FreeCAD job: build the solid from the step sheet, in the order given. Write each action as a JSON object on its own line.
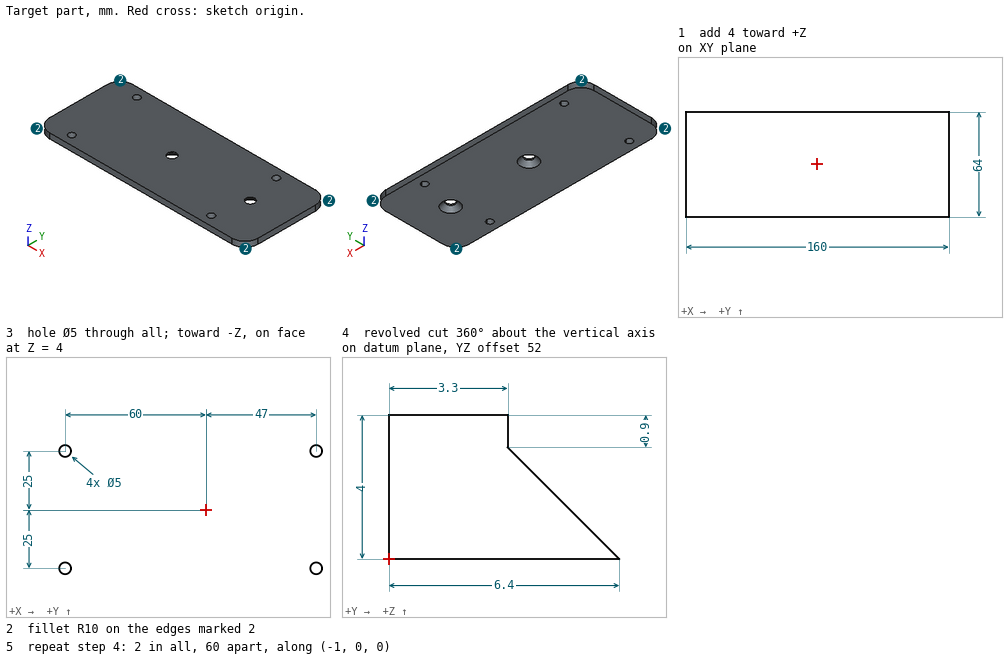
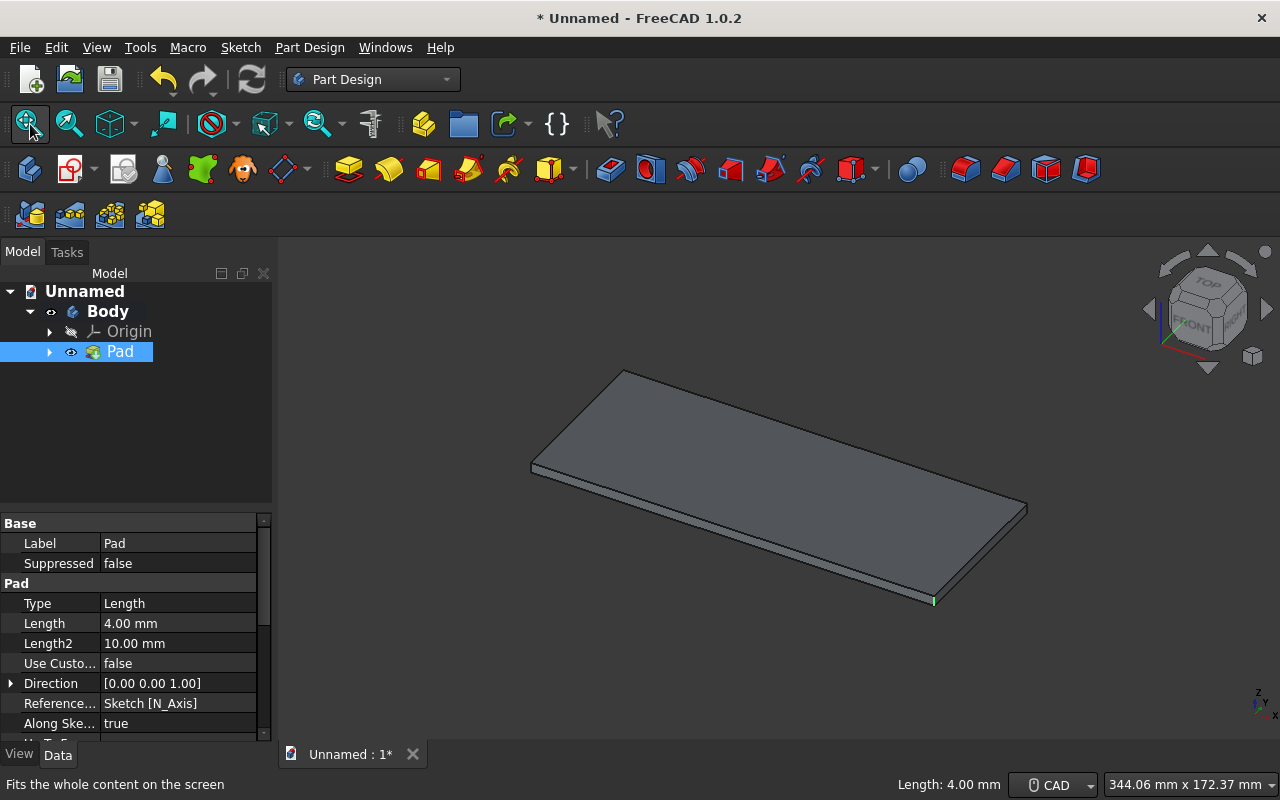
{"action": "key", "text": "0"}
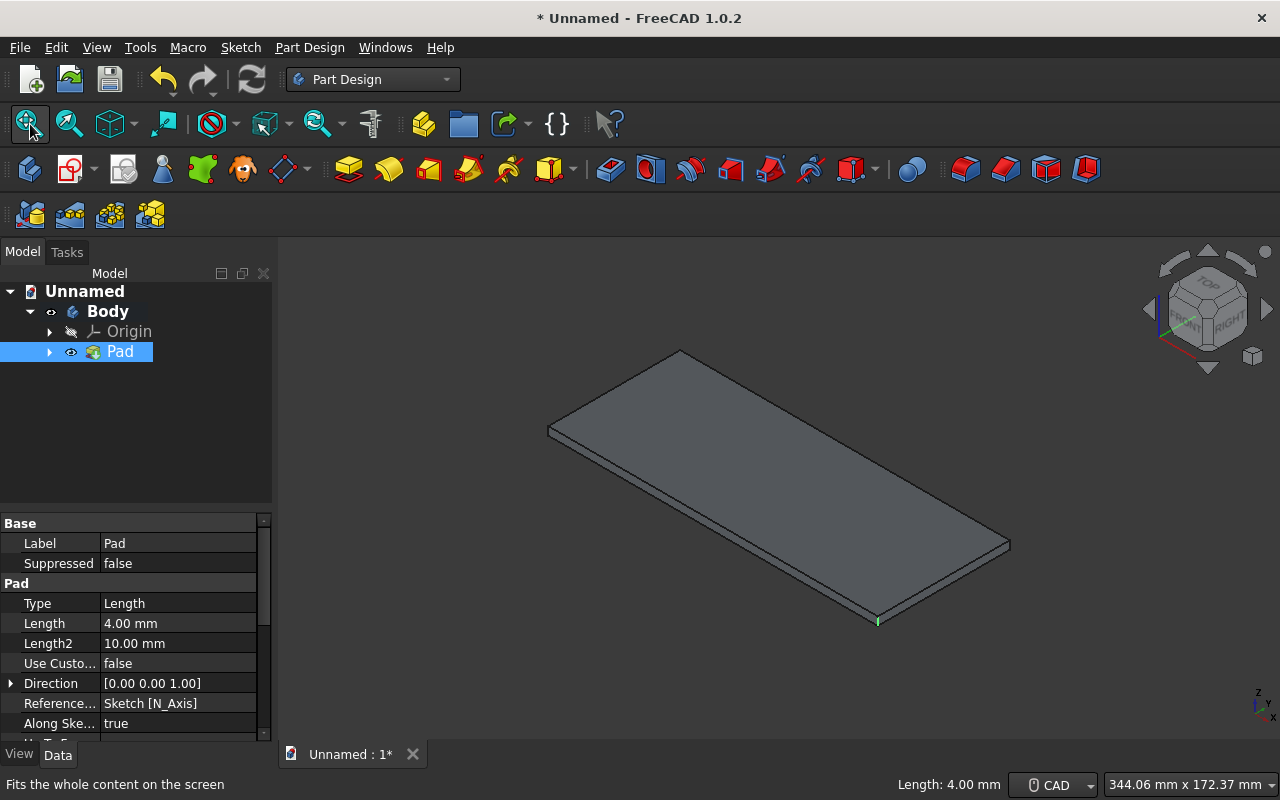
{"action": "scroll", "coordinate": [548, 430], "scroll_direction": "up", "scroll_amount": 7}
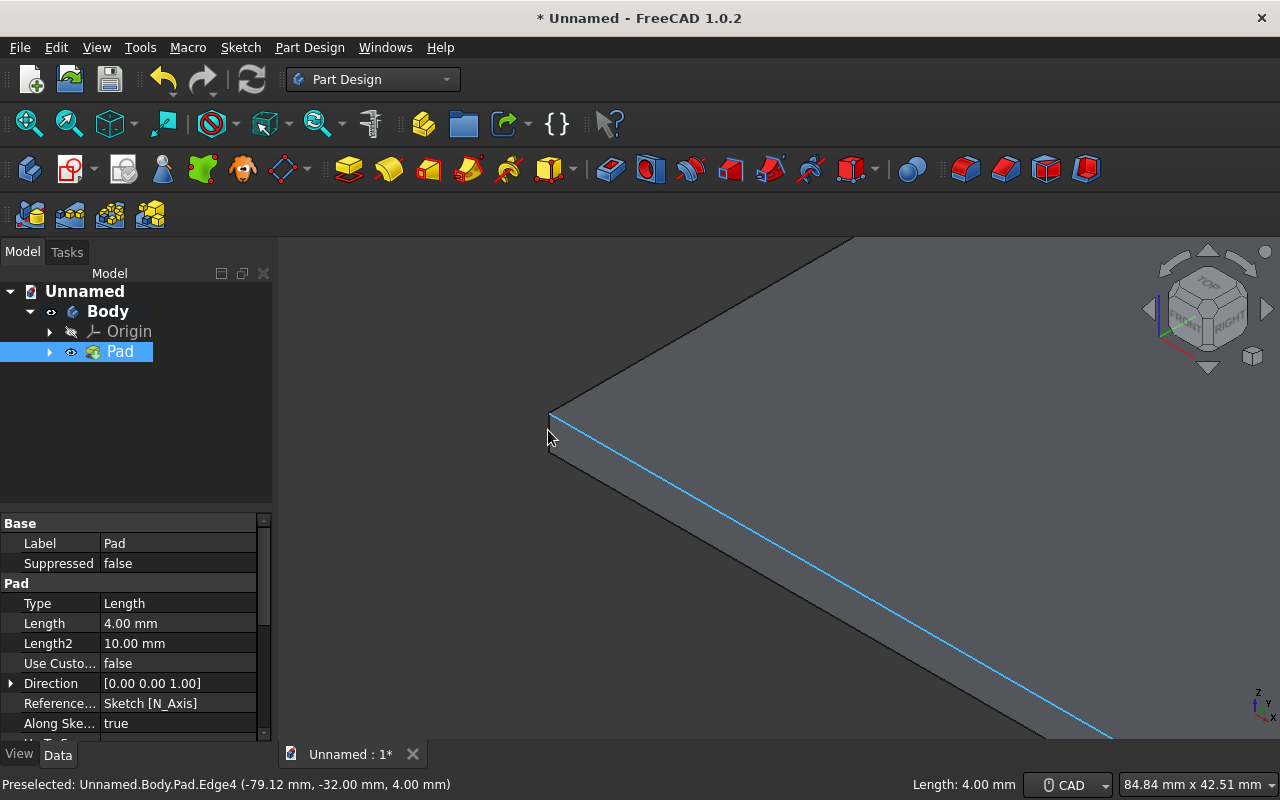
{"action": "left_click", "coordinate": [30, 124]}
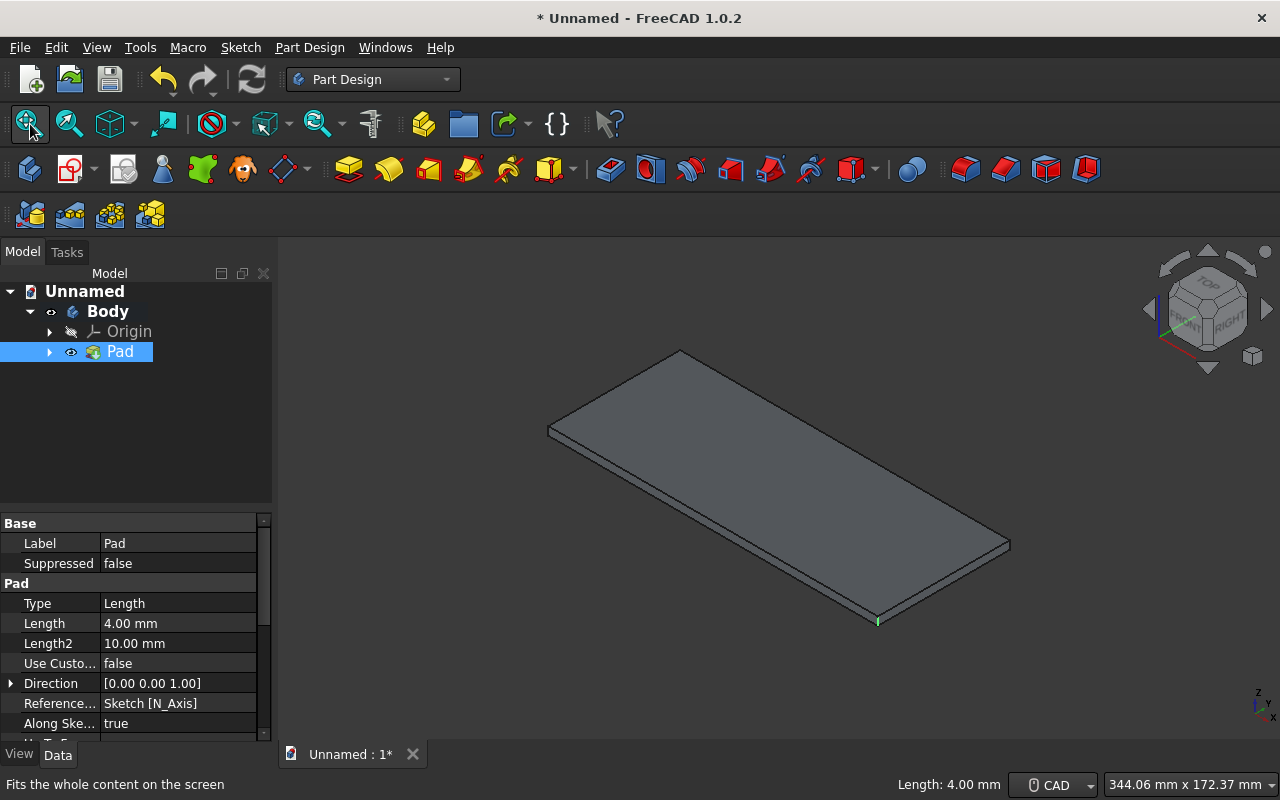
{"action": "key", "text": "2"}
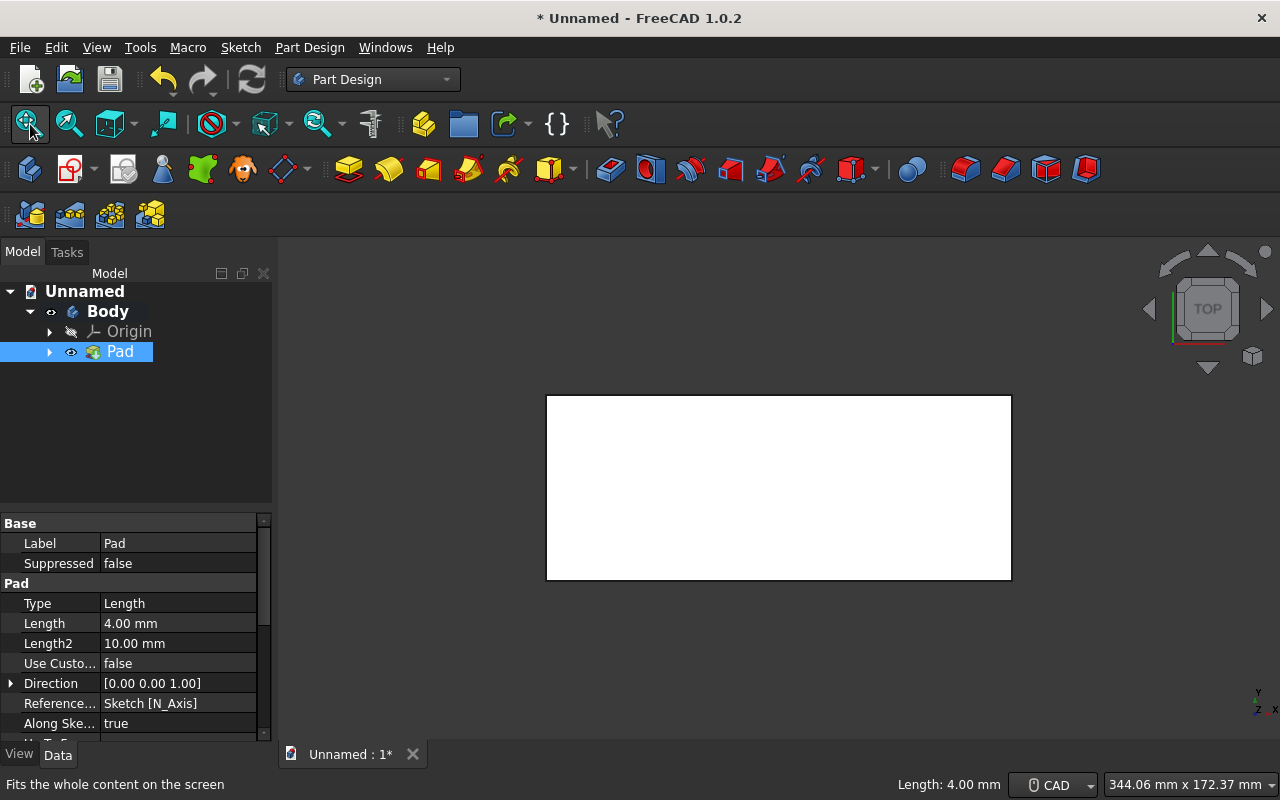
{"action": "scroll", "coordinate": [546, 580], "scroll_direction": "up", "scroll_amount": 7}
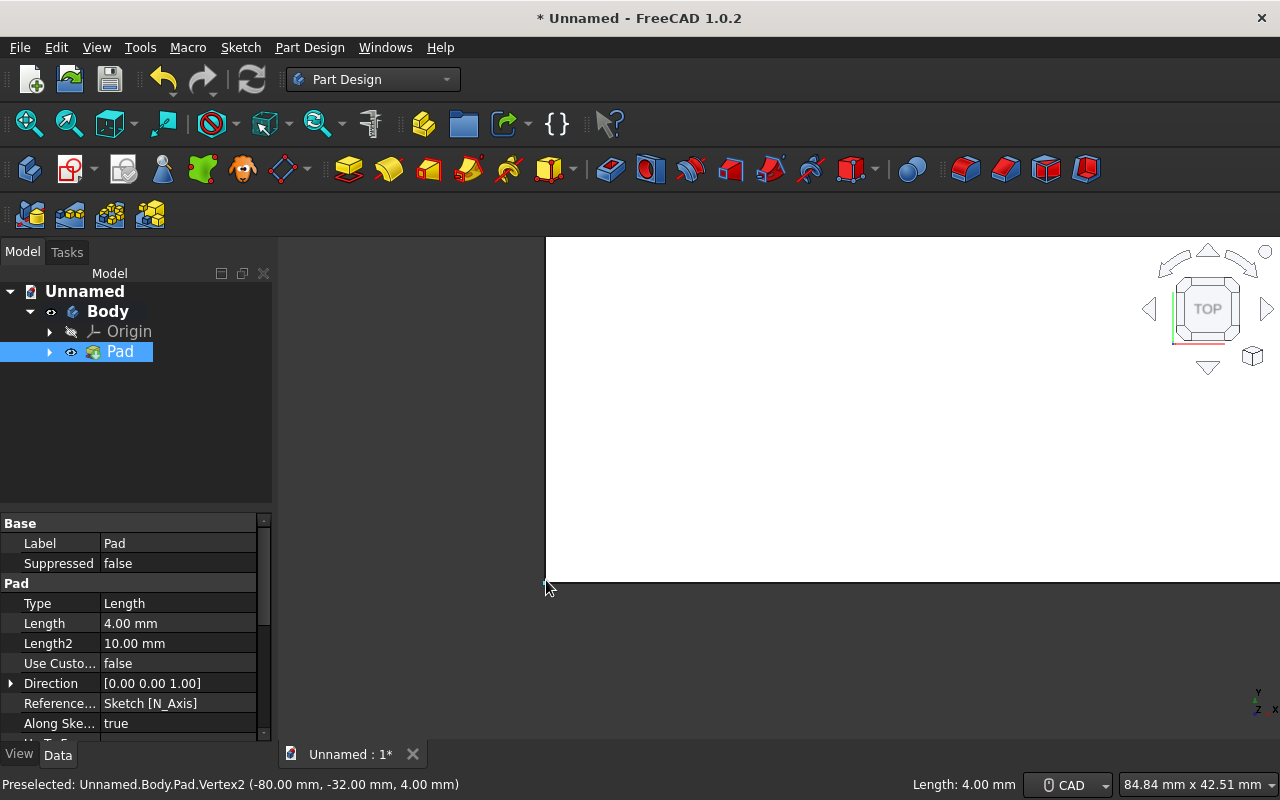
{"action": "left_click", "coordinate": [30, 124]}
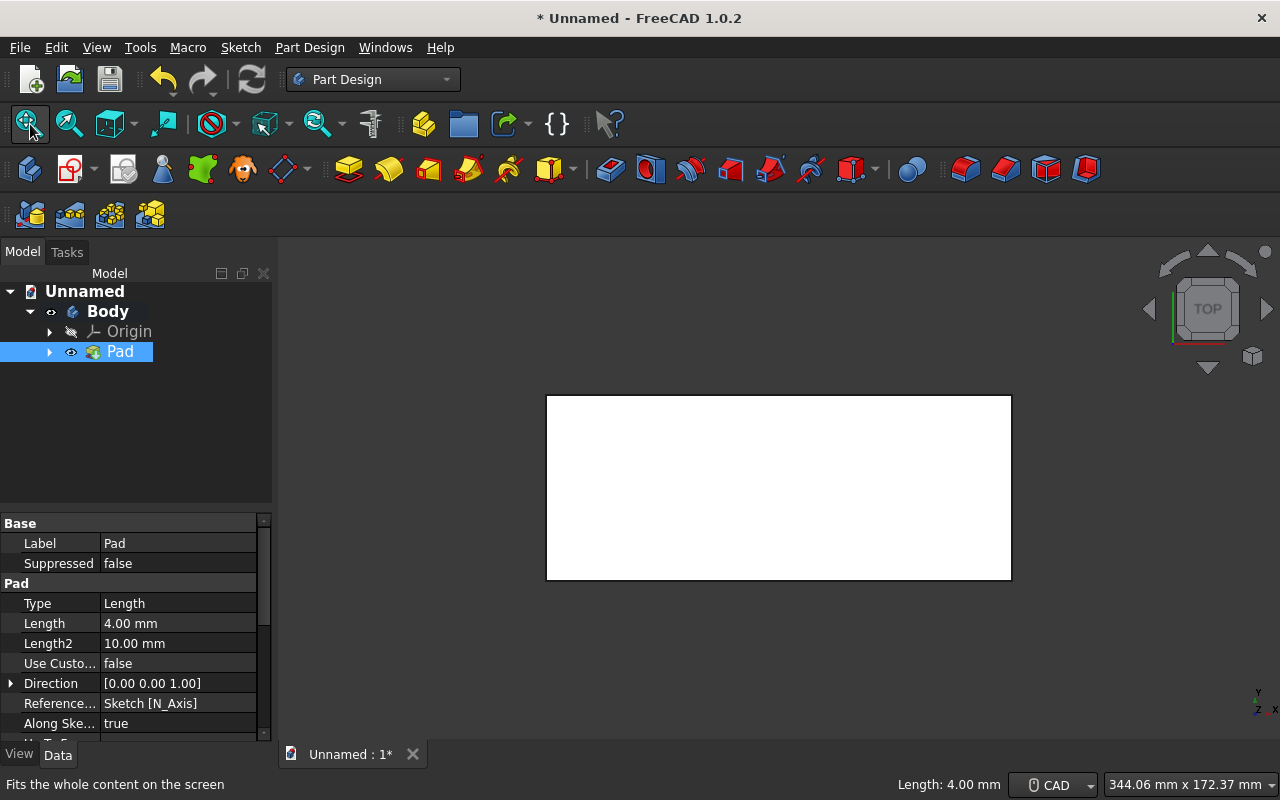
{"action": "key", "text": "1"}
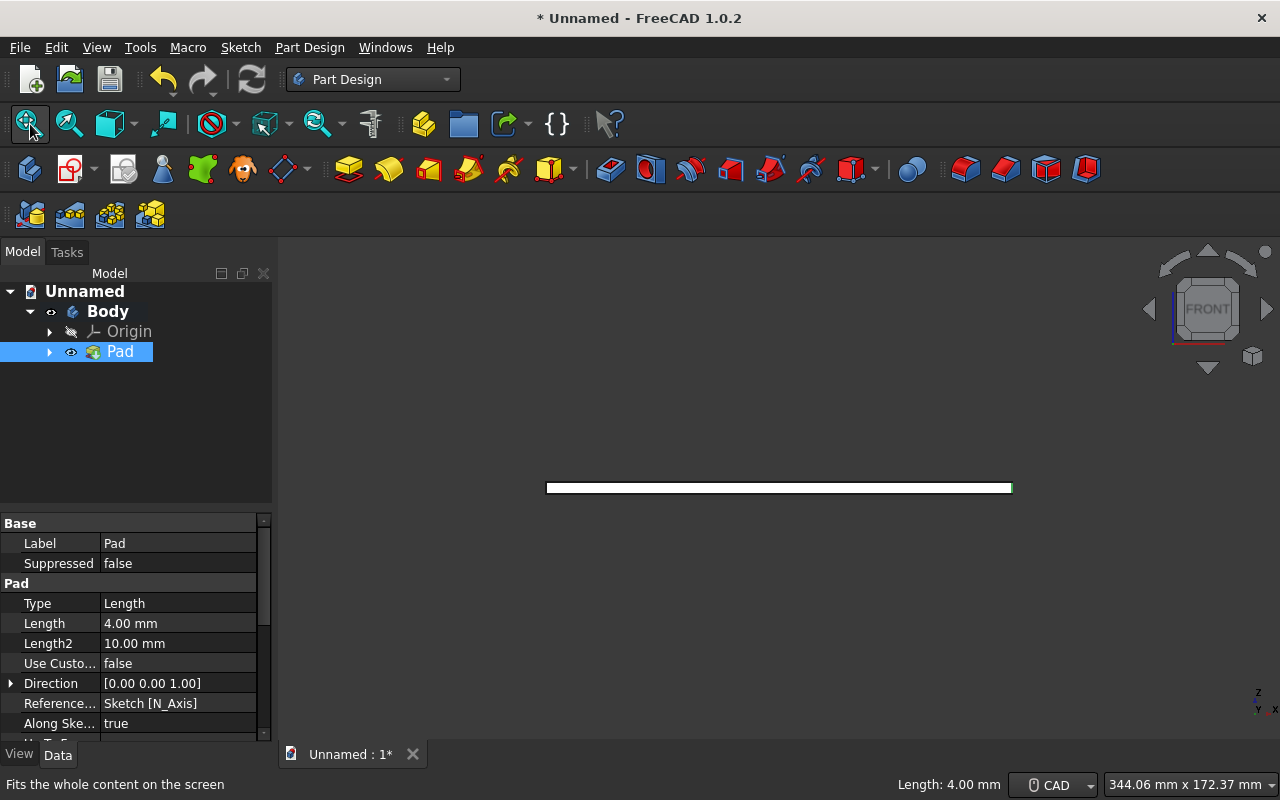
{"action": "scroll", "coordinate": [546, 487], "scroll_direction": "up", "scroll_amount": 7}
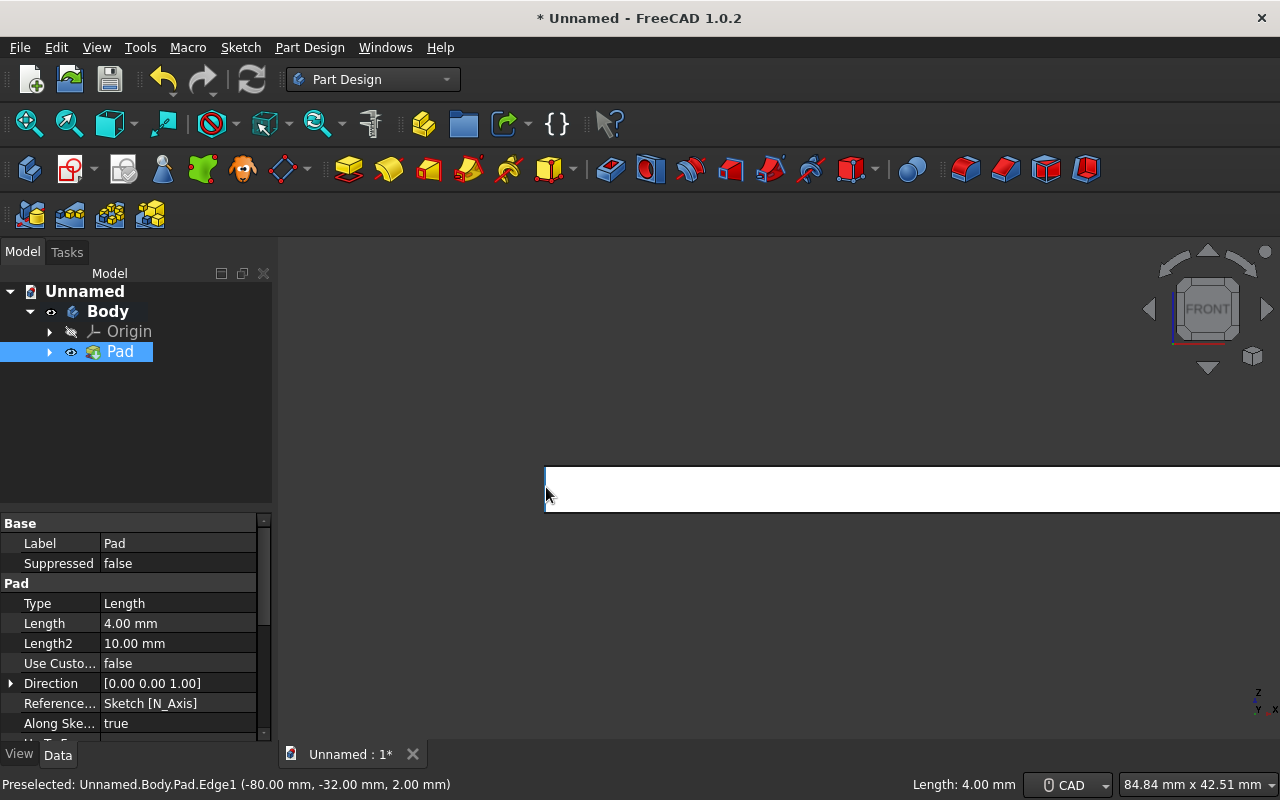
{"action": "left_click", "coordinate": [545, 489], "text": "ctrl"}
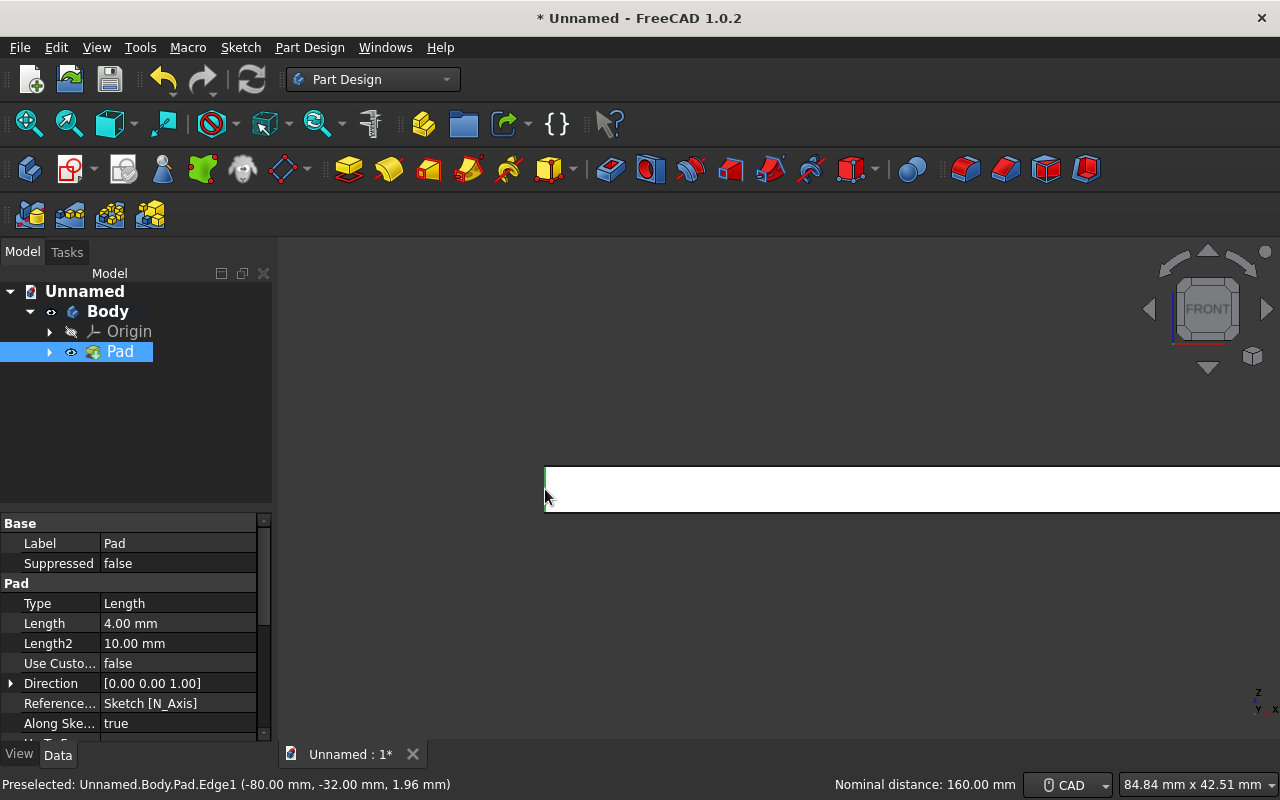
{"action": "left_click", "coordinate": [30, 124]}